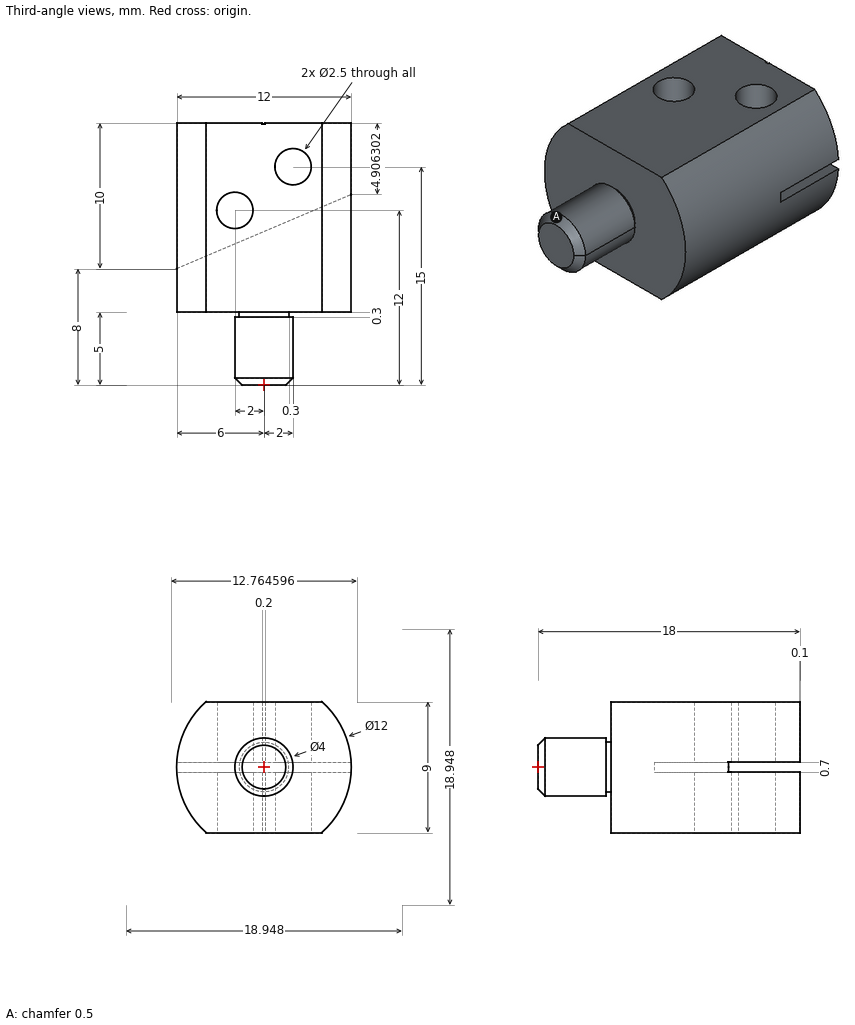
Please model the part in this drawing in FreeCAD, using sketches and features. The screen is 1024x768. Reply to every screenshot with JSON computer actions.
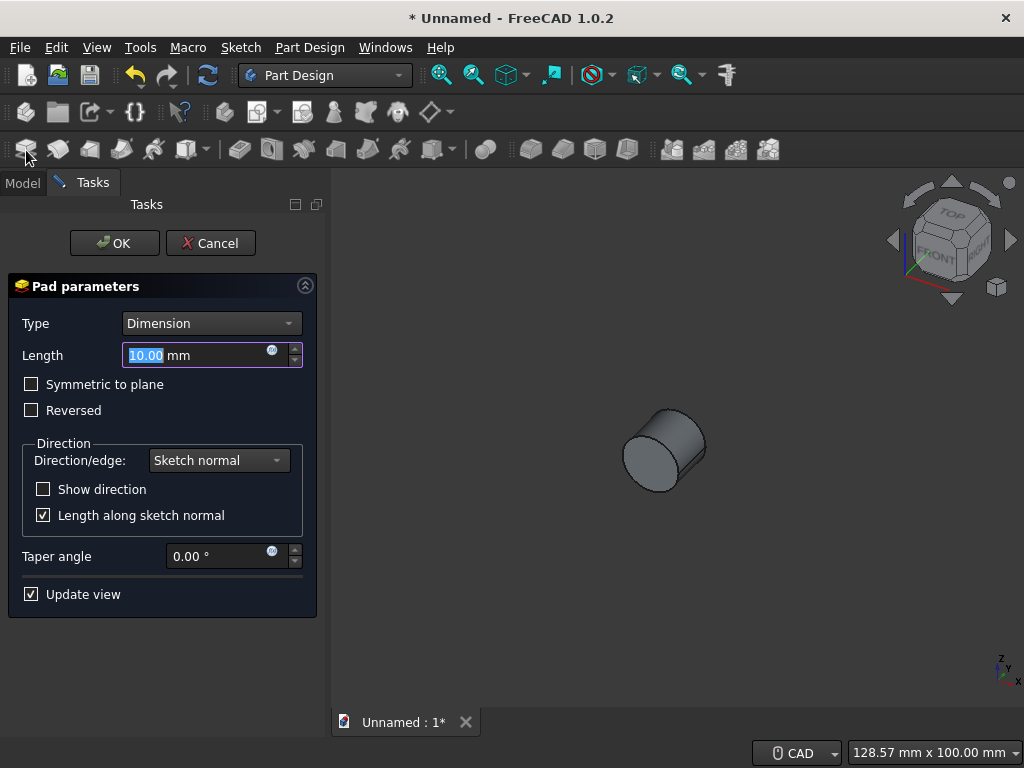
{"action": "type", "text": "18"}
{"action": "key", "text": "Tab"}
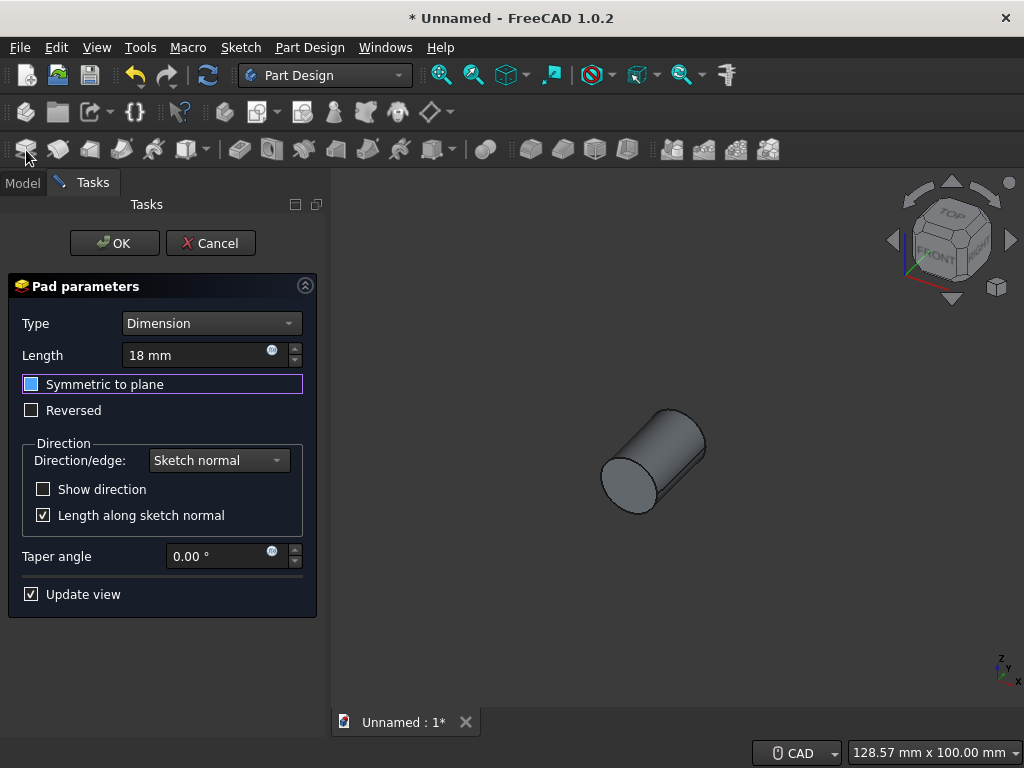
{"action": "left_click", "coordinate": [30, 410]}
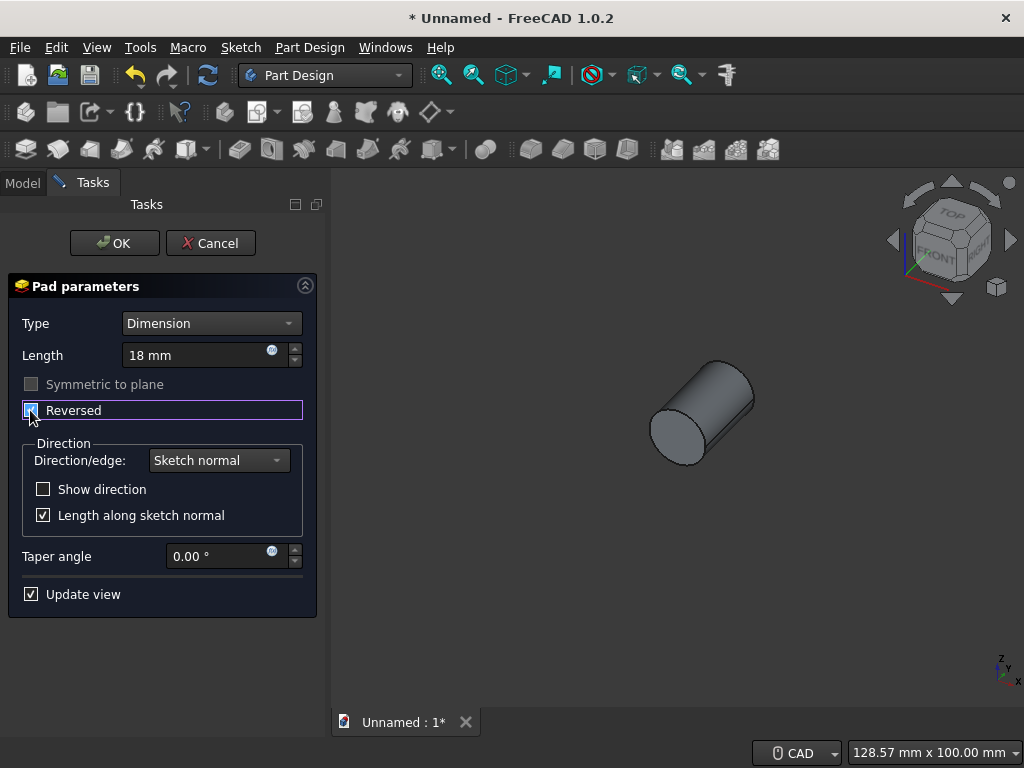
{"action": "left_click", "coordinate": [115, 243]}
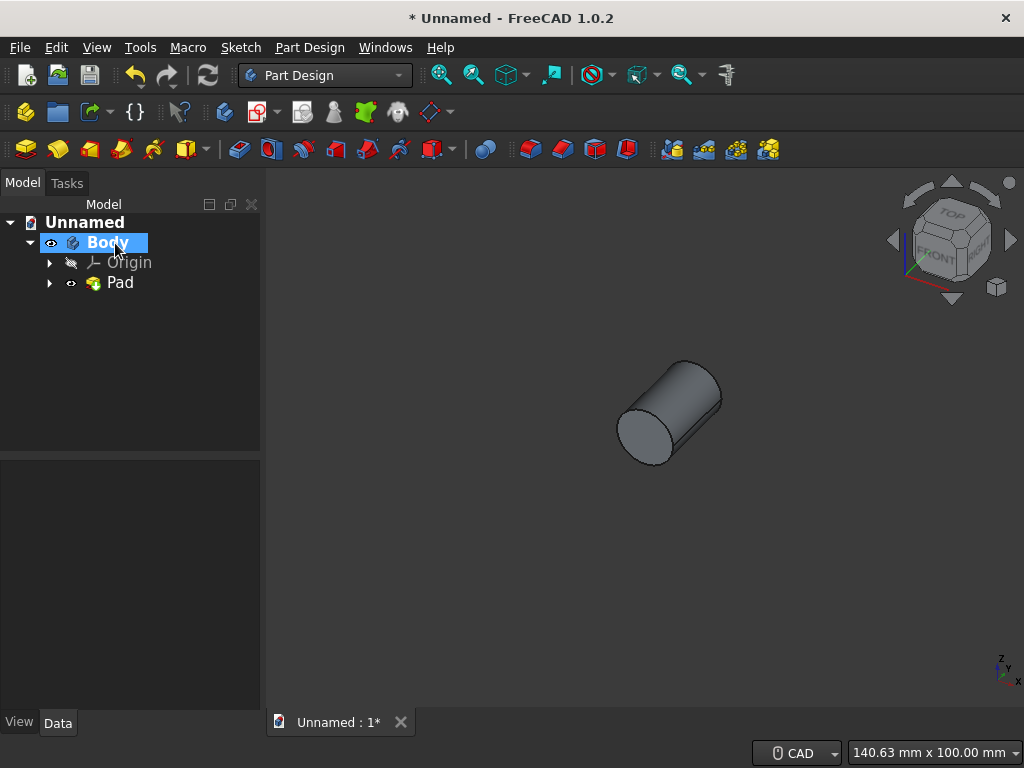
{"action": "key", "text": "v f"}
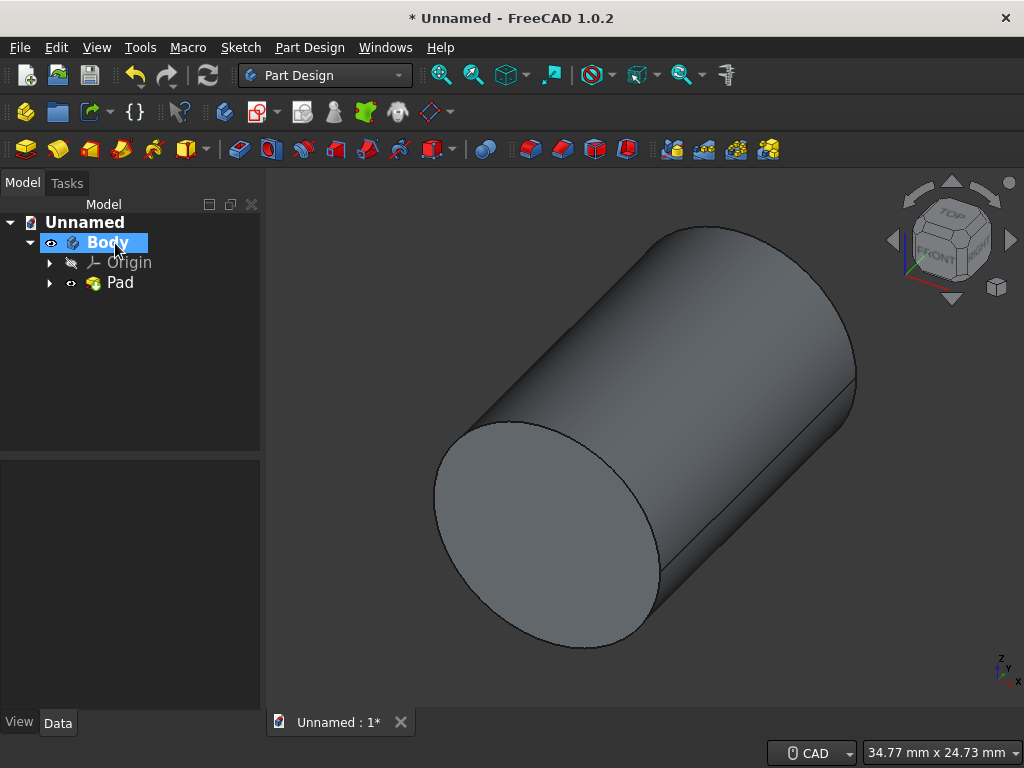
{"action": "left_click", "coordinate": [547, 534]}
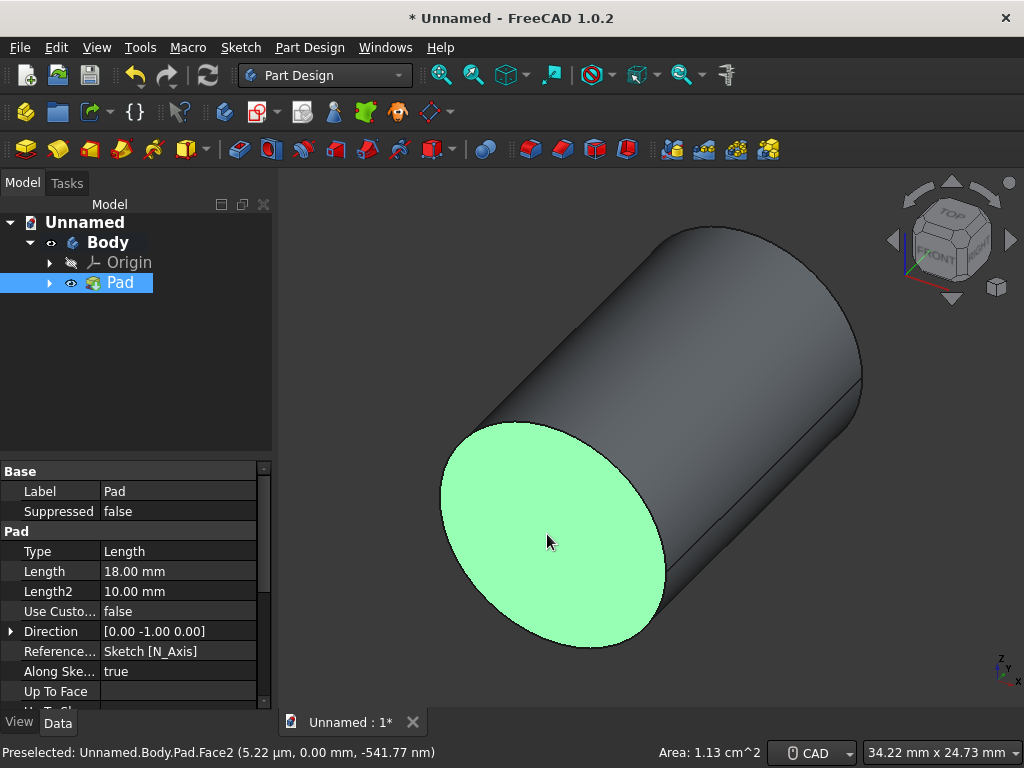
{"action": "left_click", "coordinate": [258, 112]}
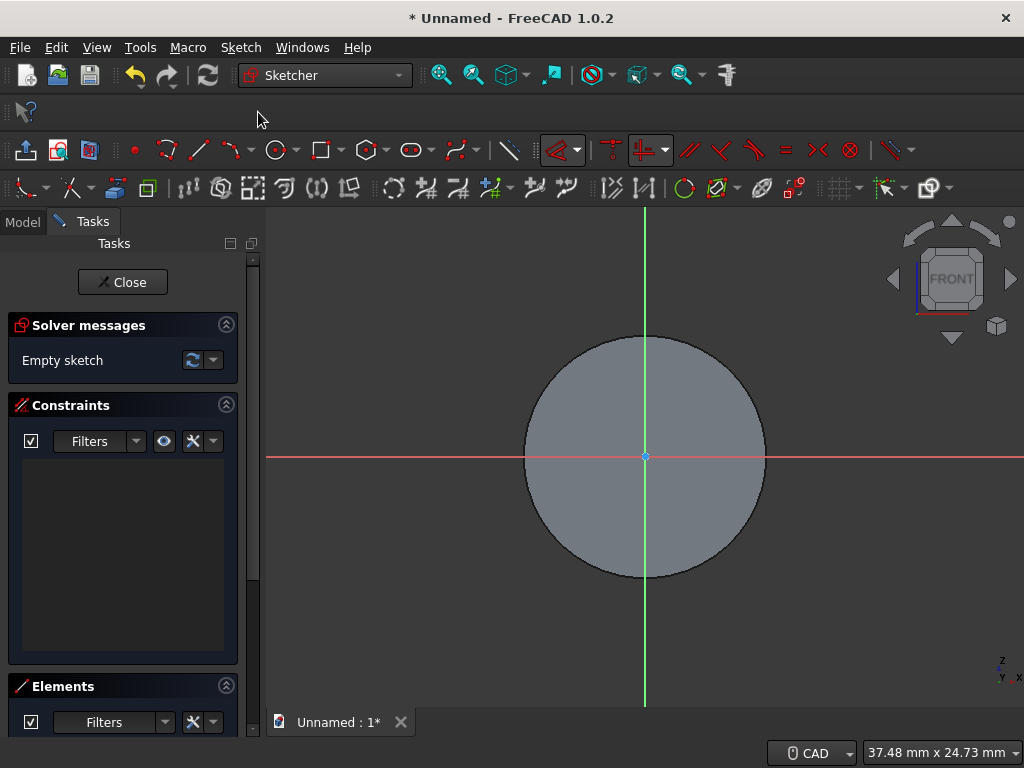
{"action": "scroll", "coordinate": [294, 457], "scroll_direction": "down", "scroll_amount": 1}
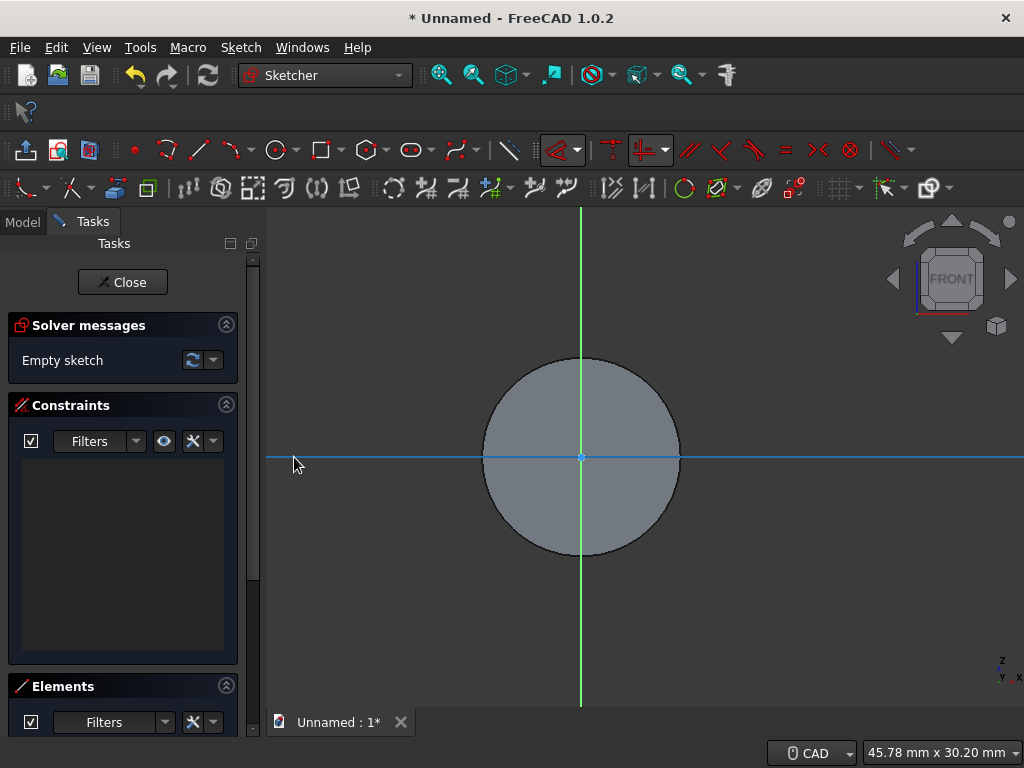
{"action": "left_click", "coordinate": [344, 150]}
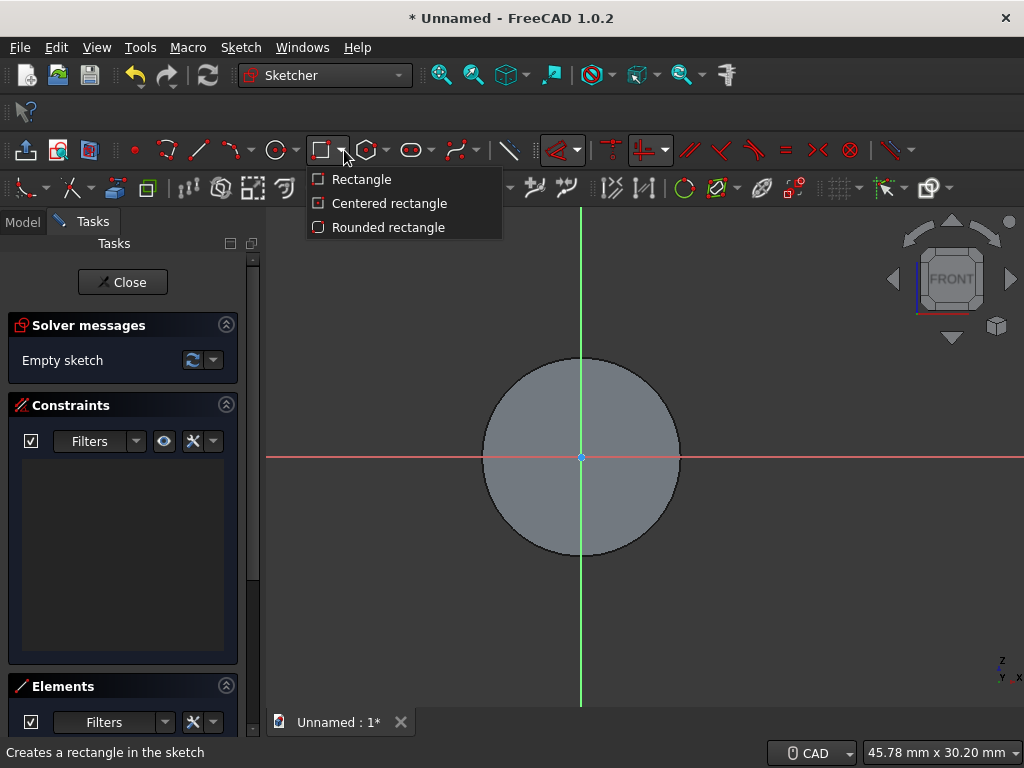
{"action": "left_click", "coordinate": [404, 203]}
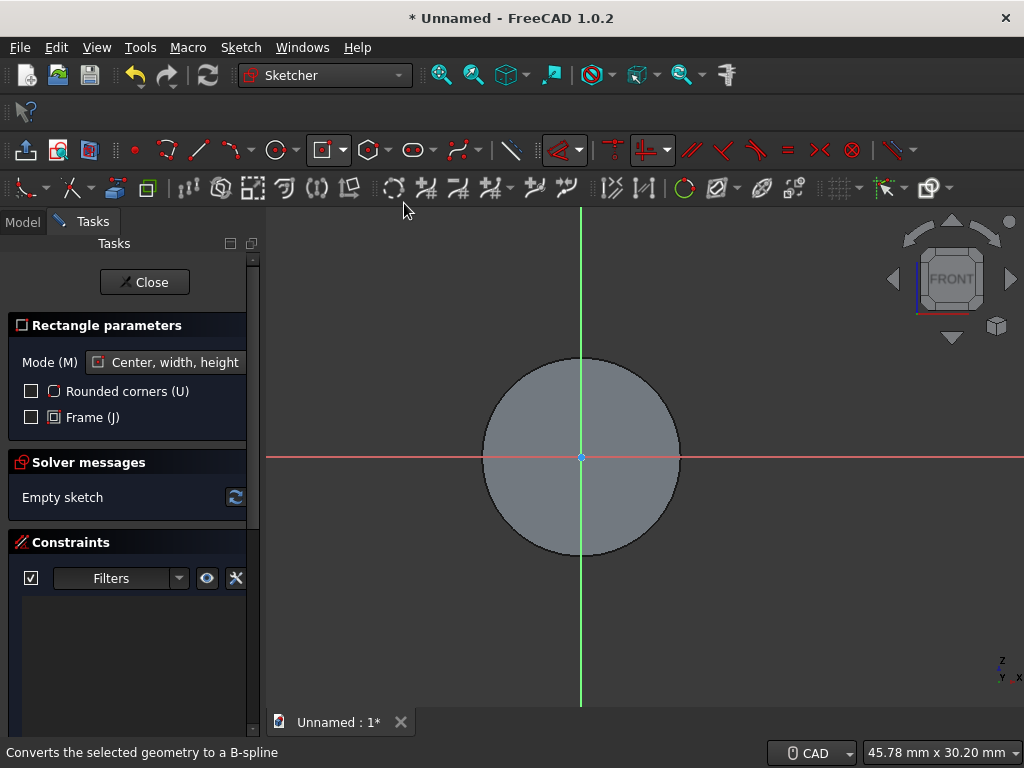
{"action": "left_click", "coordinate": [581, 457]}
{"action": "left_click", "coordinate": [738, 300]}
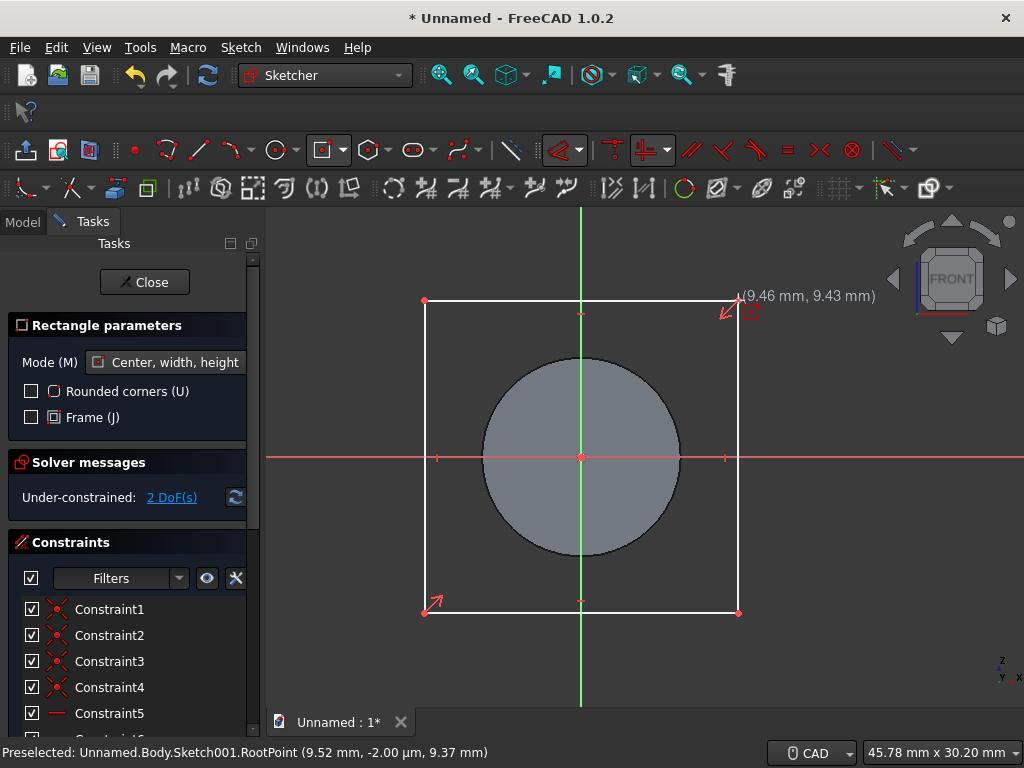
{"action": "left_click", "coordinate": [276, 150]}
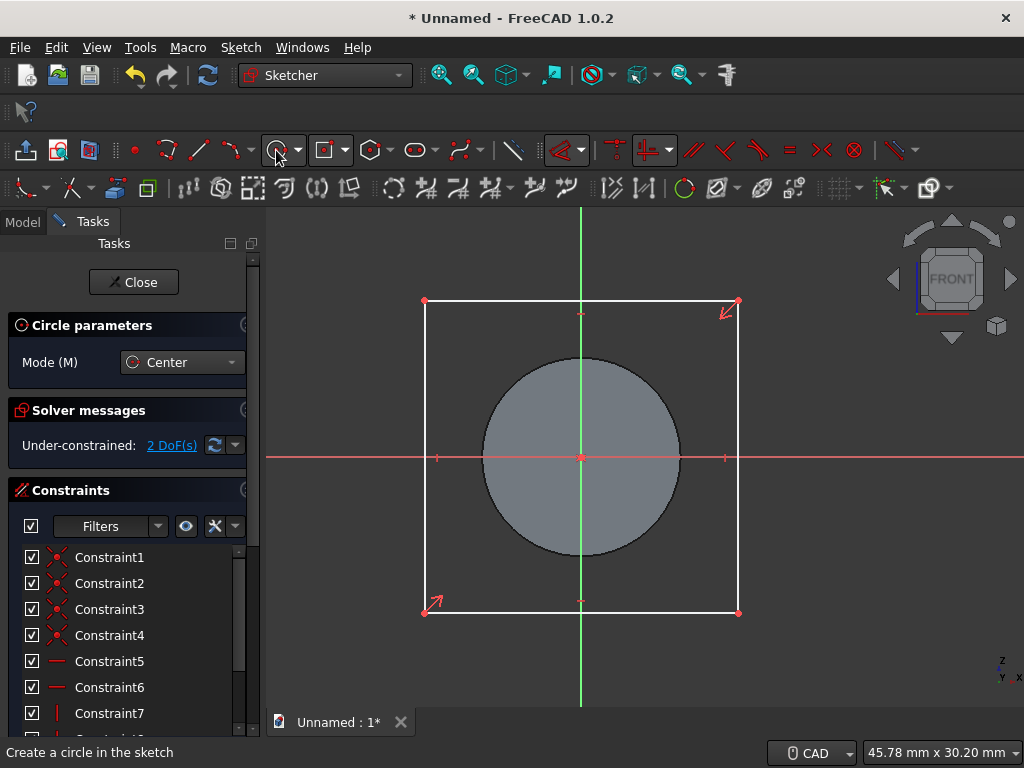
{"action": "left_click", "coordinate": [581, 457]}
{"action": "left_click", "coordinate": [605, 434]}
{"action": "key", "text": "Escape"}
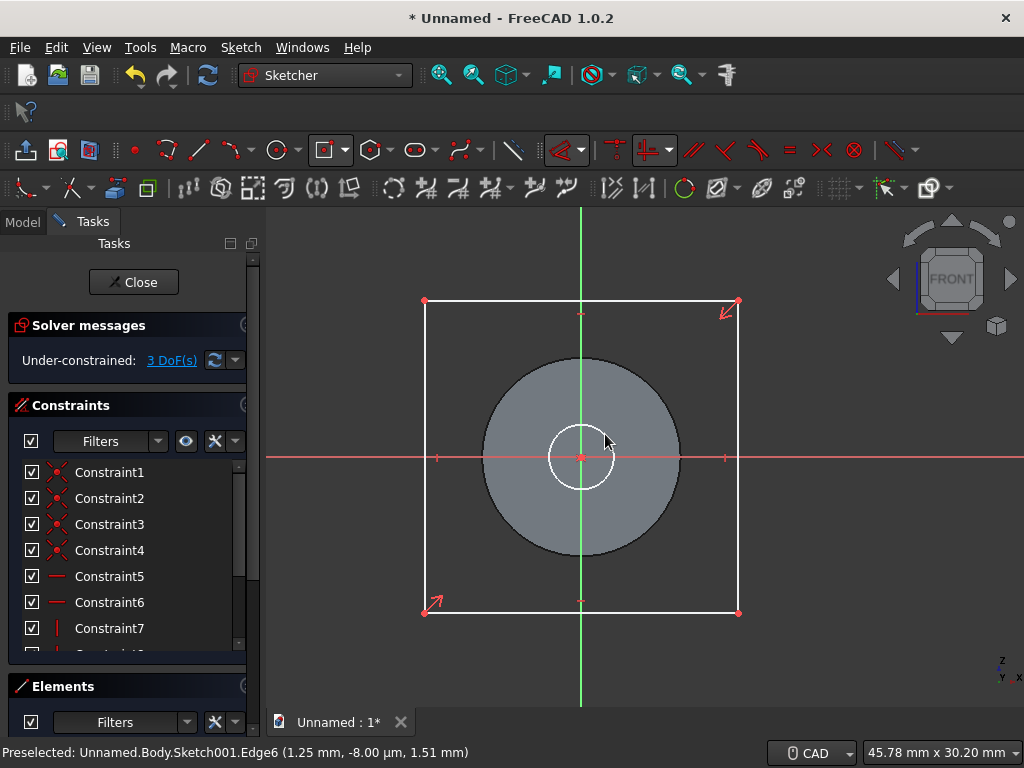
{"action": "left_click", "coordinate": [604, 434]}